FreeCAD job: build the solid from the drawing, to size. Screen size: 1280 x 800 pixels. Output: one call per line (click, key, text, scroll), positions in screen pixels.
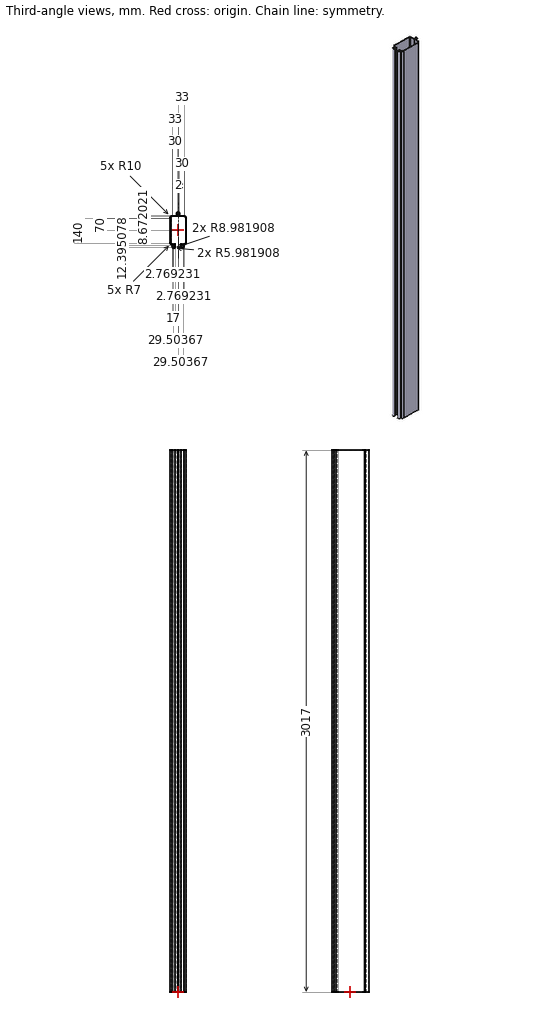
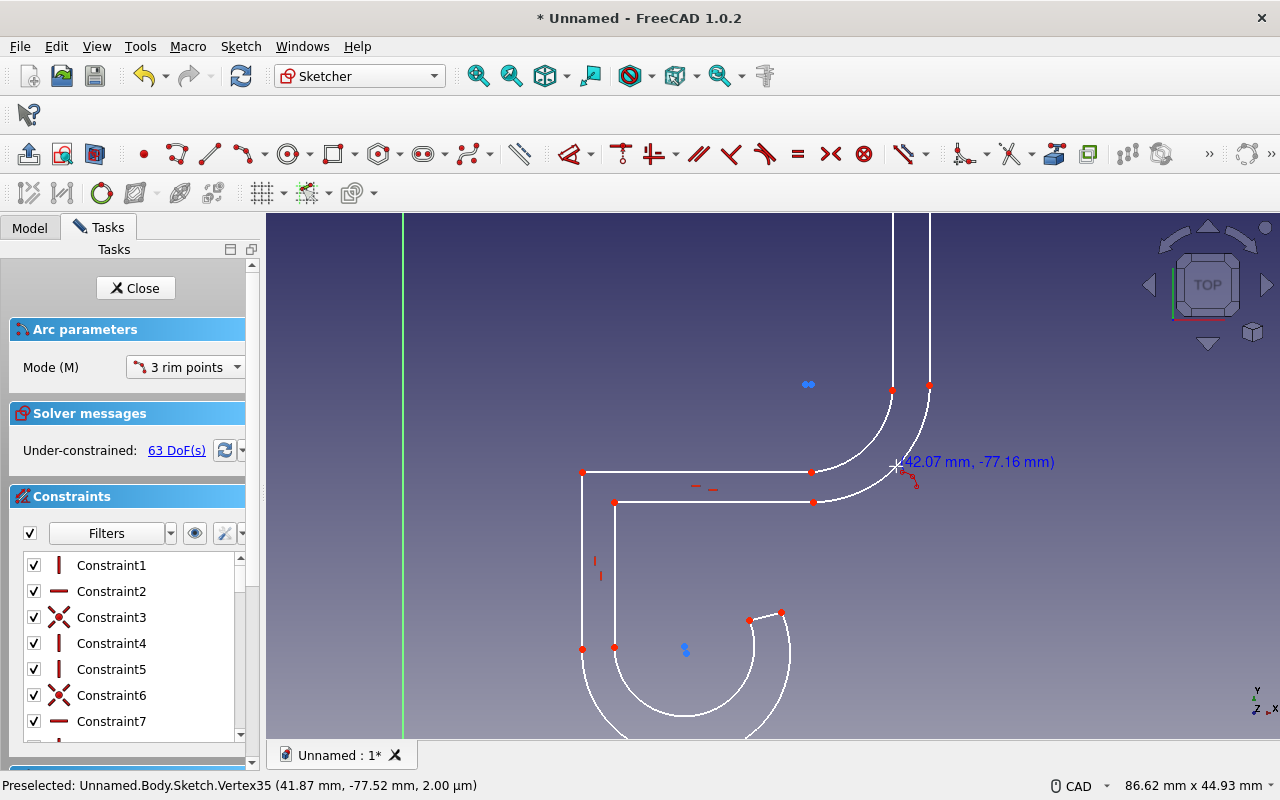
scroll(752, 620, down, 10)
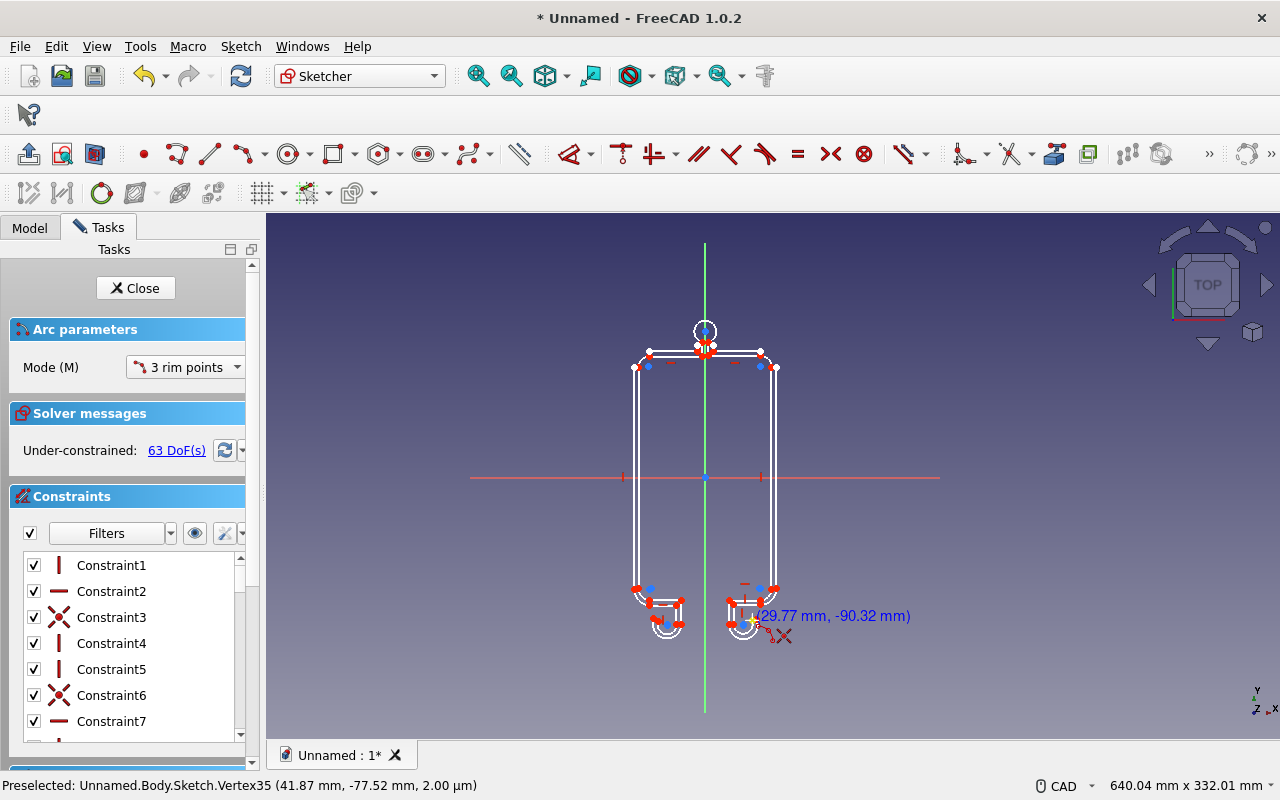
scroll(777, 367, up, 7)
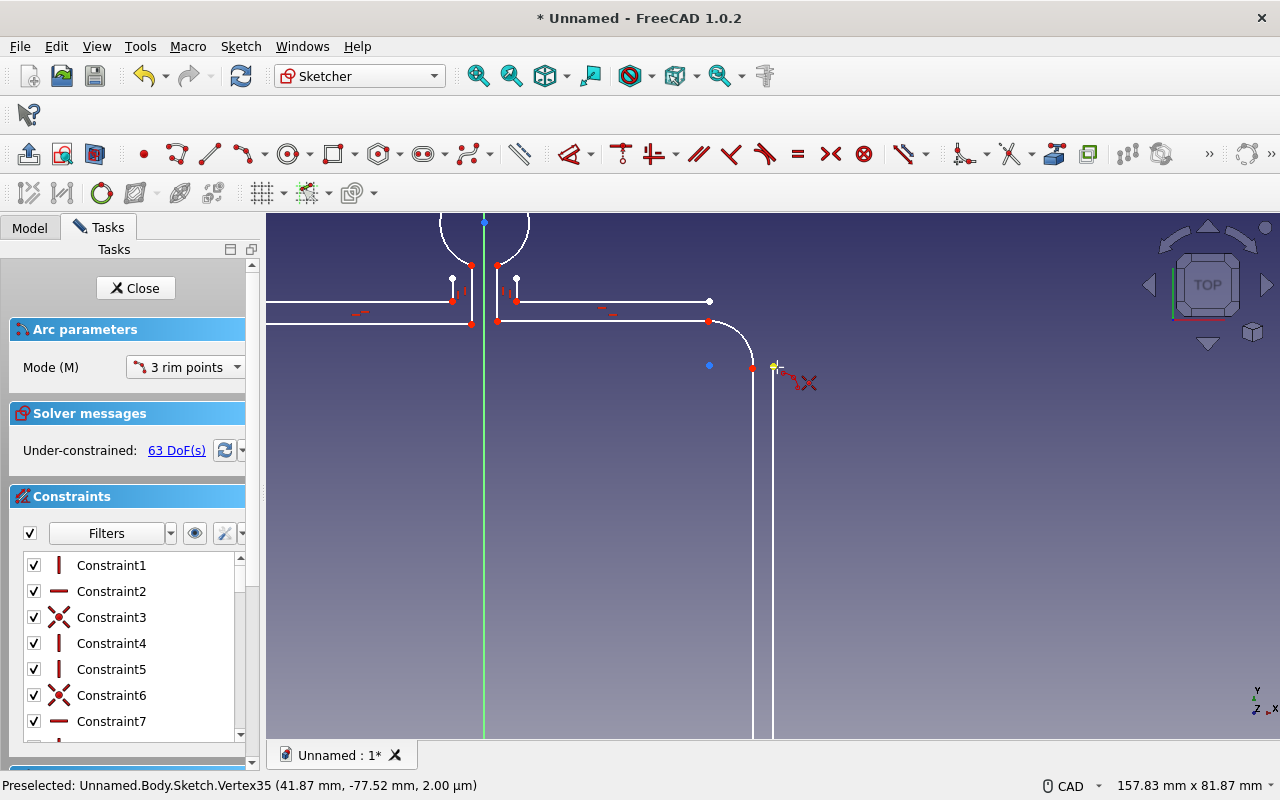
click(773, 367)
click(710, 302)
click(755, 320)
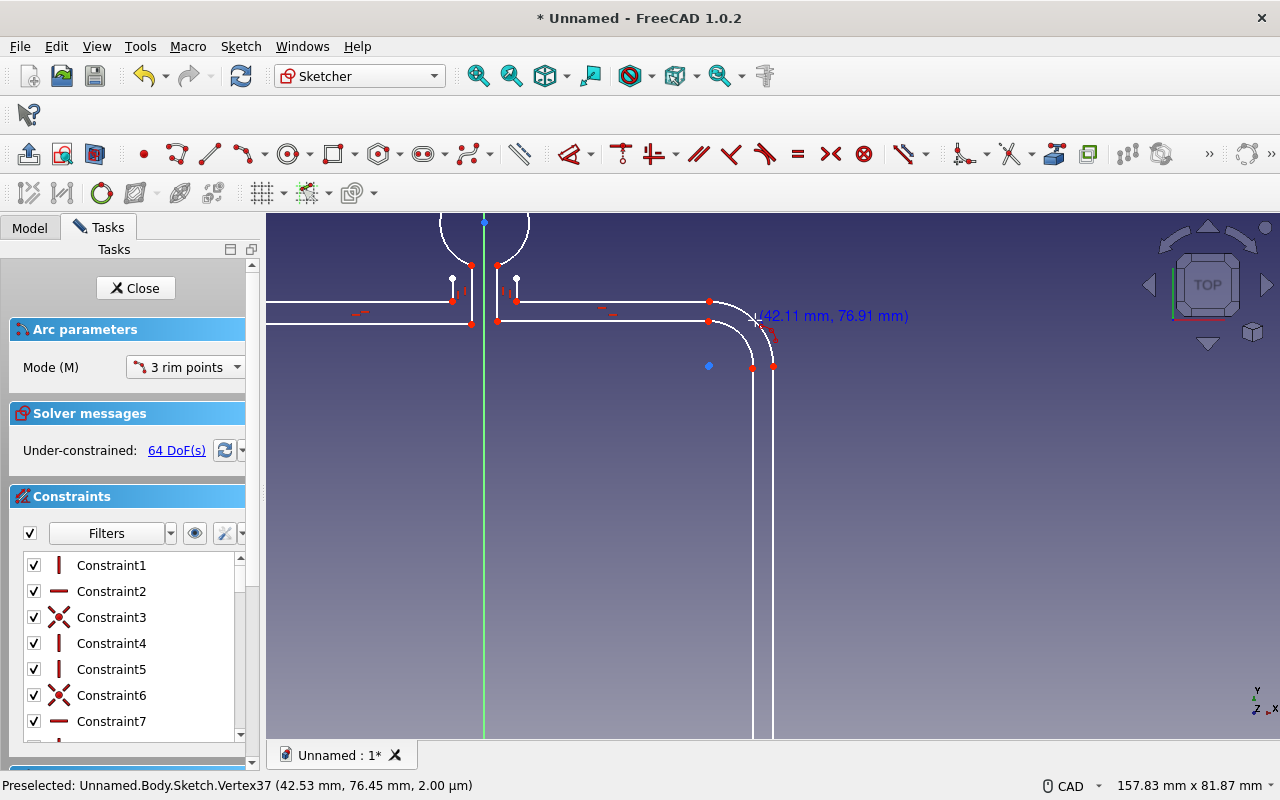
scroll(517, 277, up, 2)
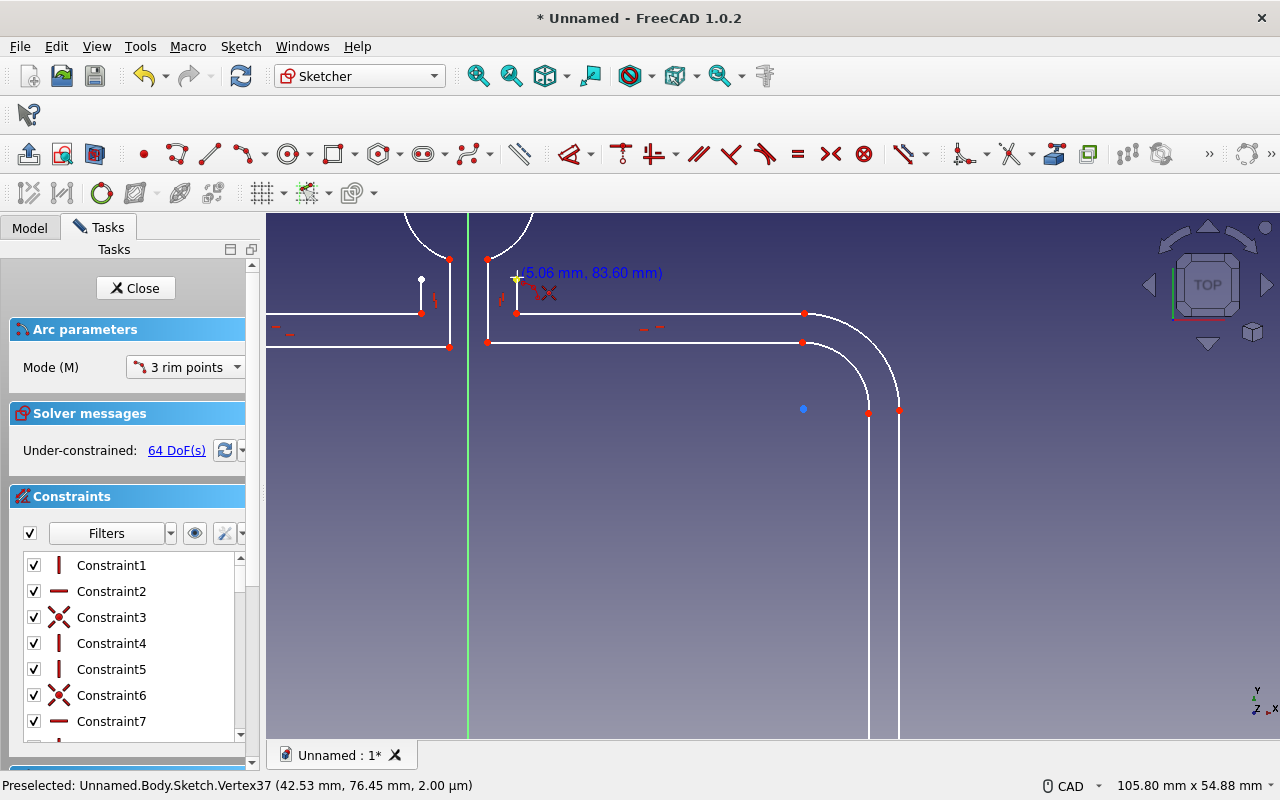
click(517, 279)
click(421, 279)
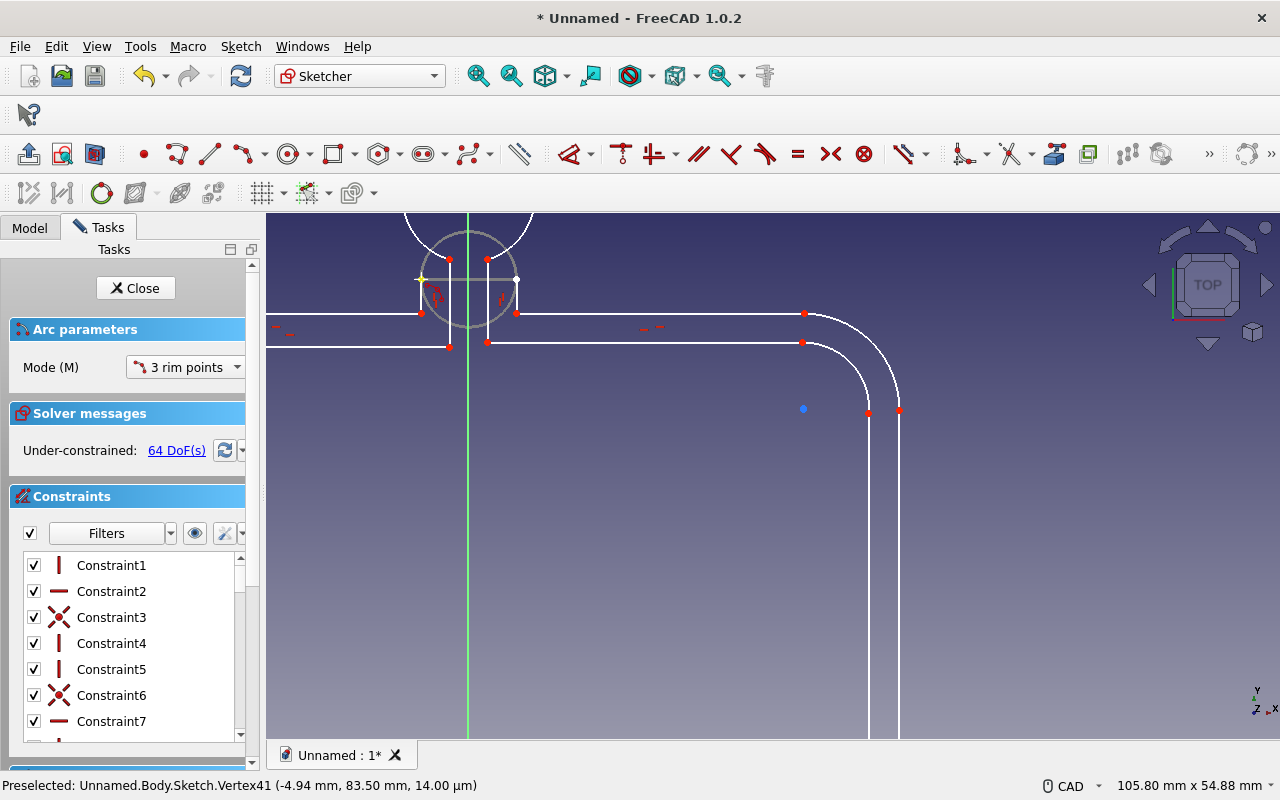
scroll(751, 358, down, 9)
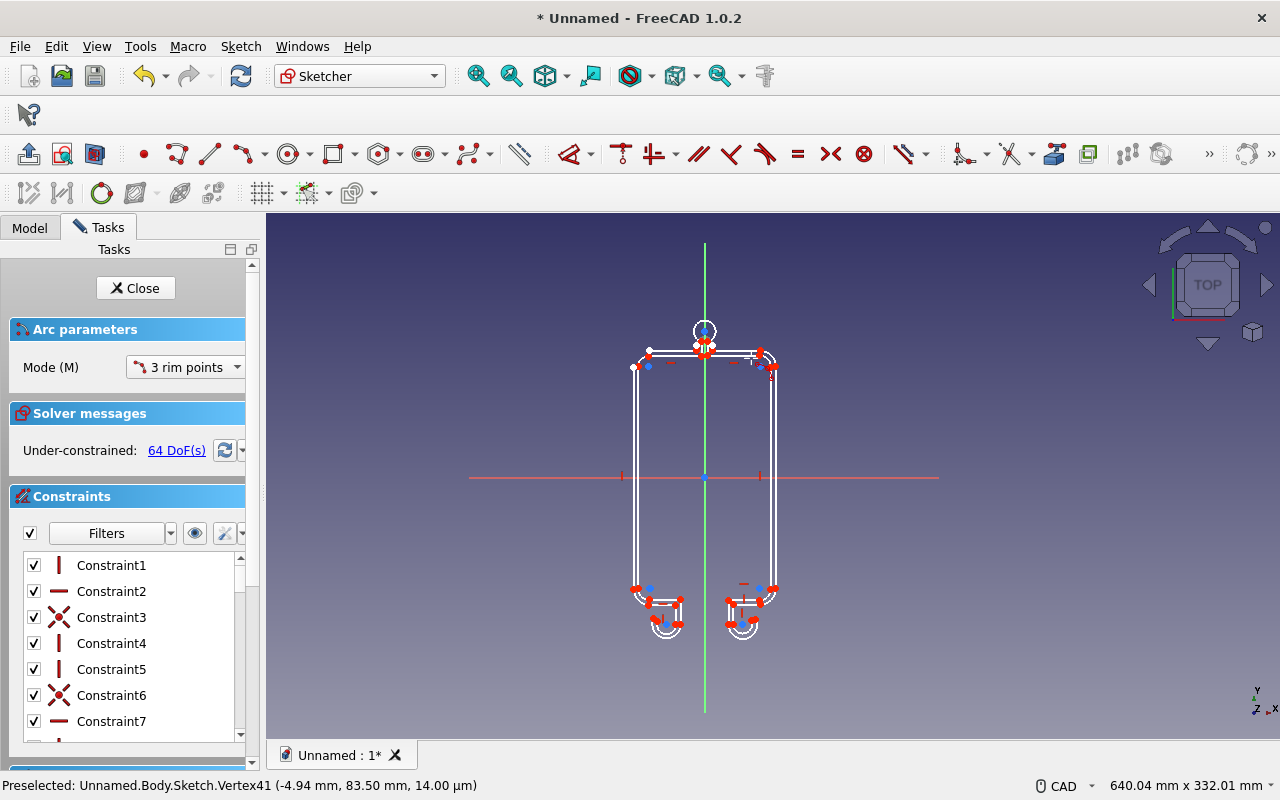
scroll(713, 317, up, 7)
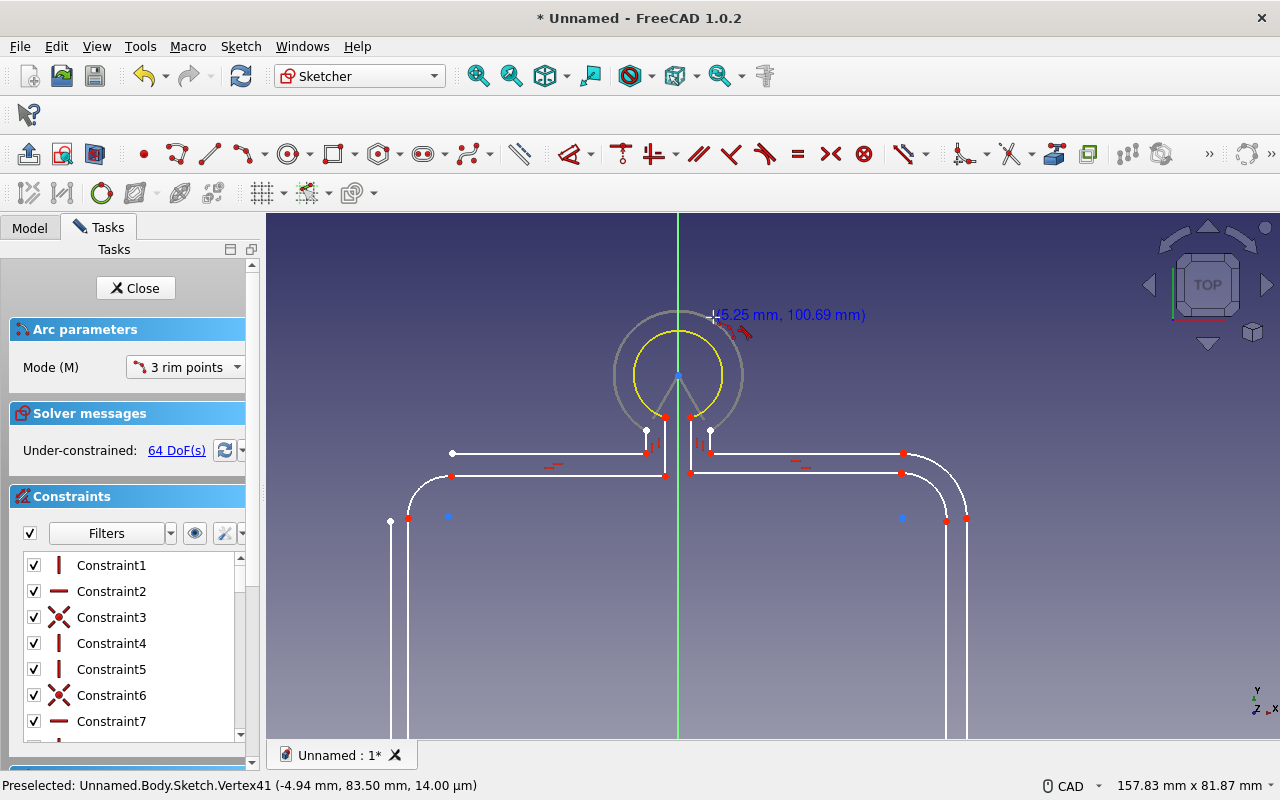
click(710, 318)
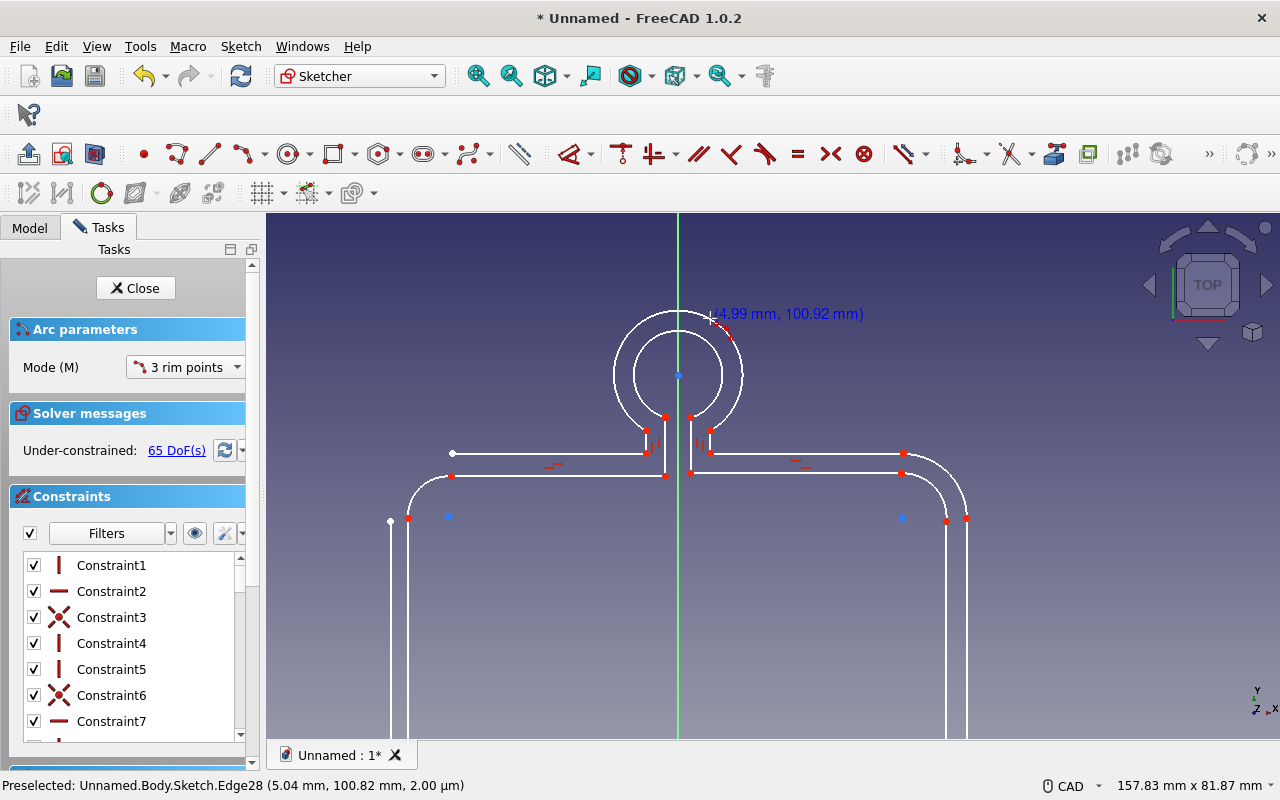
click(453, 454)
click(391, 521)
click(408, 472)
key(Escape)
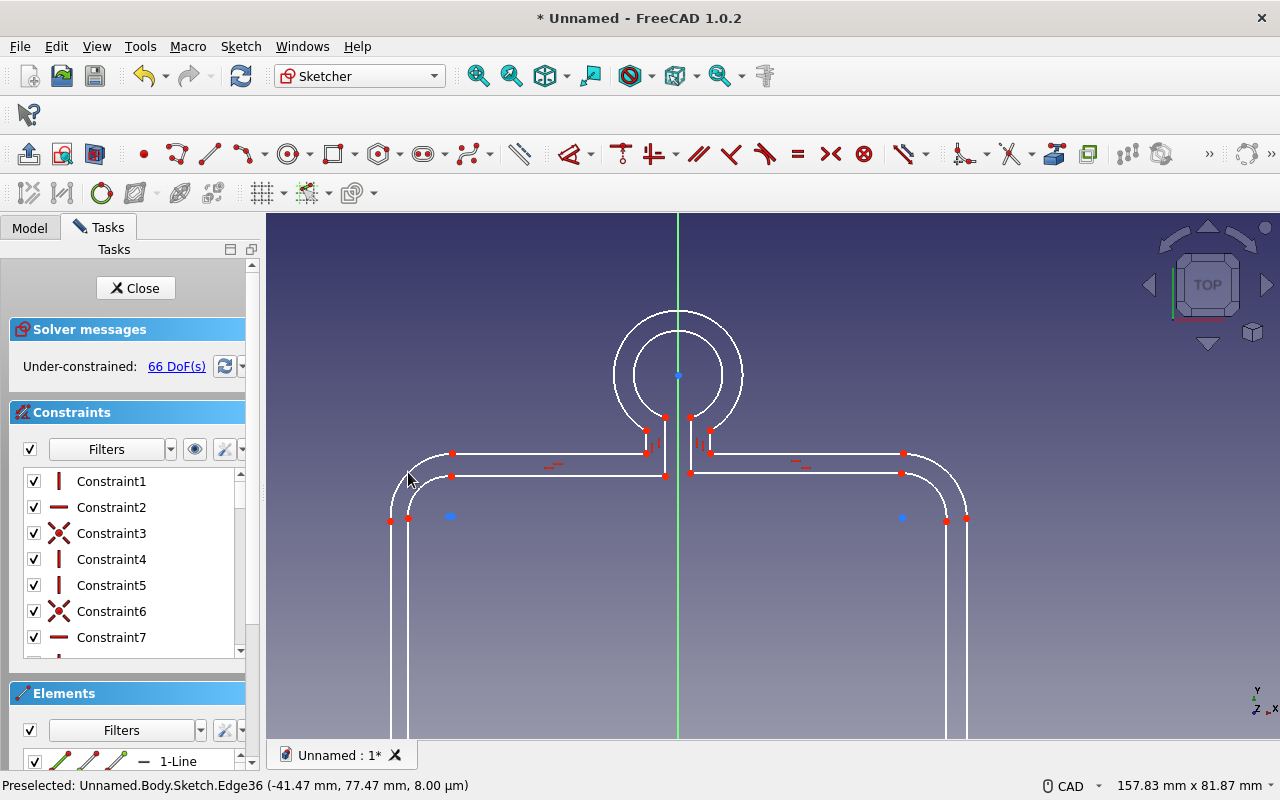
click(391, 701)